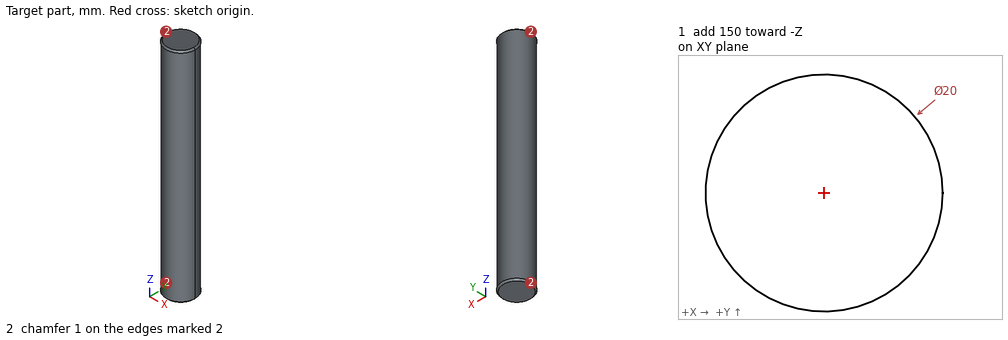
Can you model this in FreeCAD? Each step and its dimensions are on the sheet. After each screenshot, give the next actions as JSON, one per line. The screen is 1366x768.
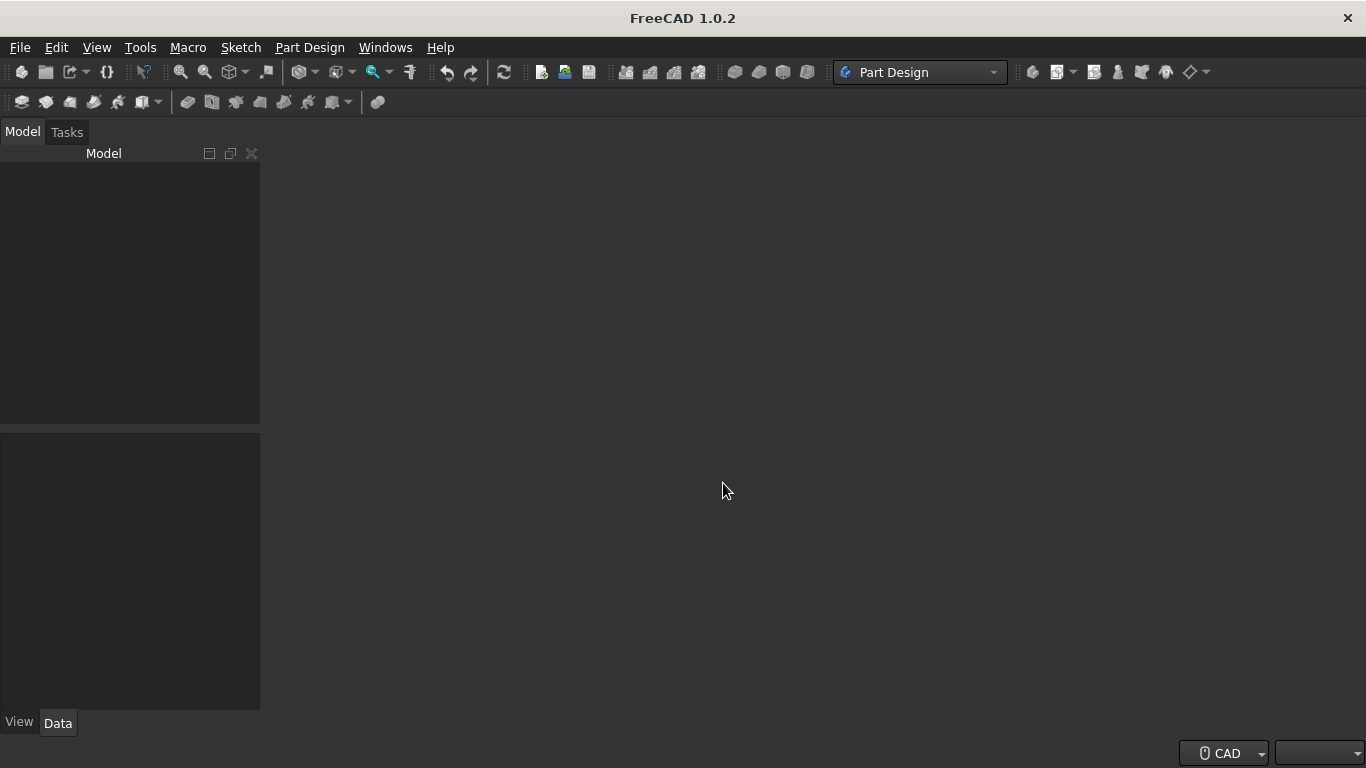
{"action": "key", "text": "ctrl+n"}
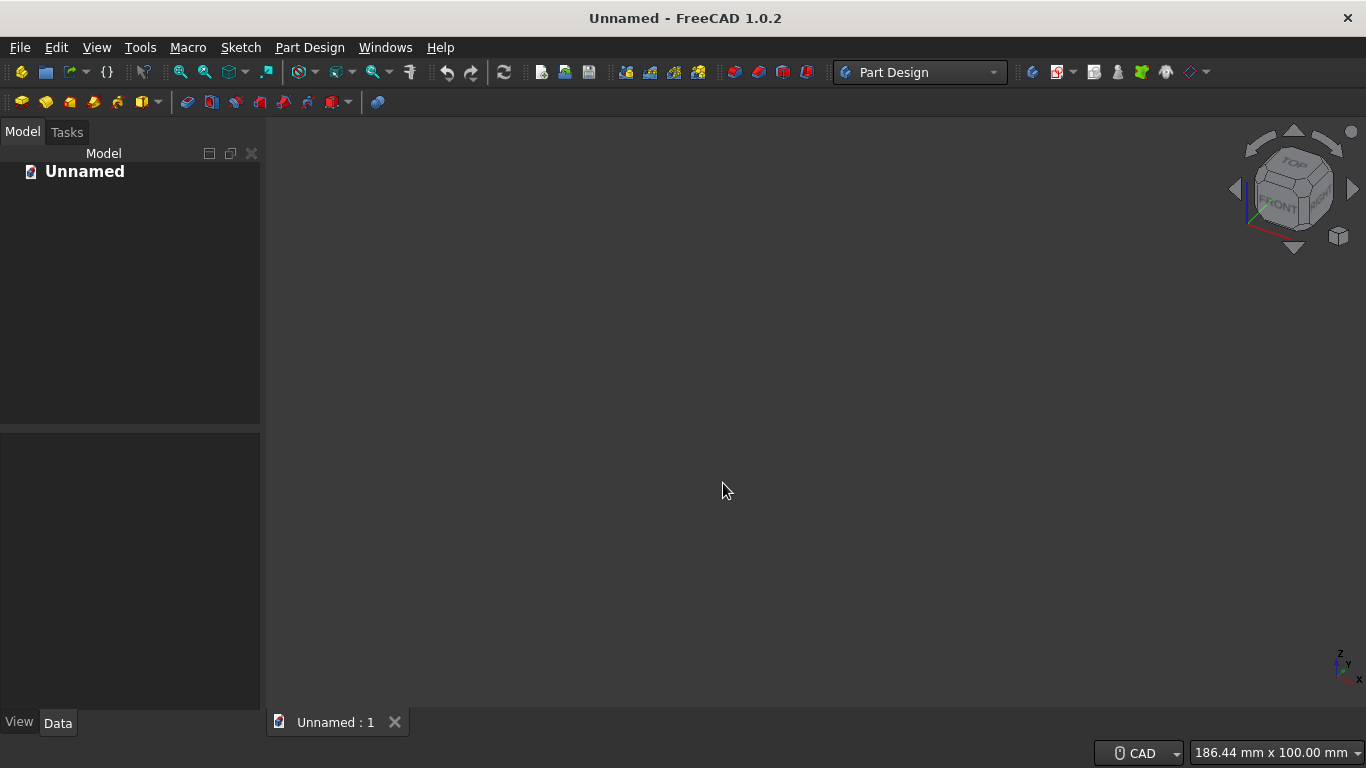
{"action": "left_click", "coordinate": [1058, 72]}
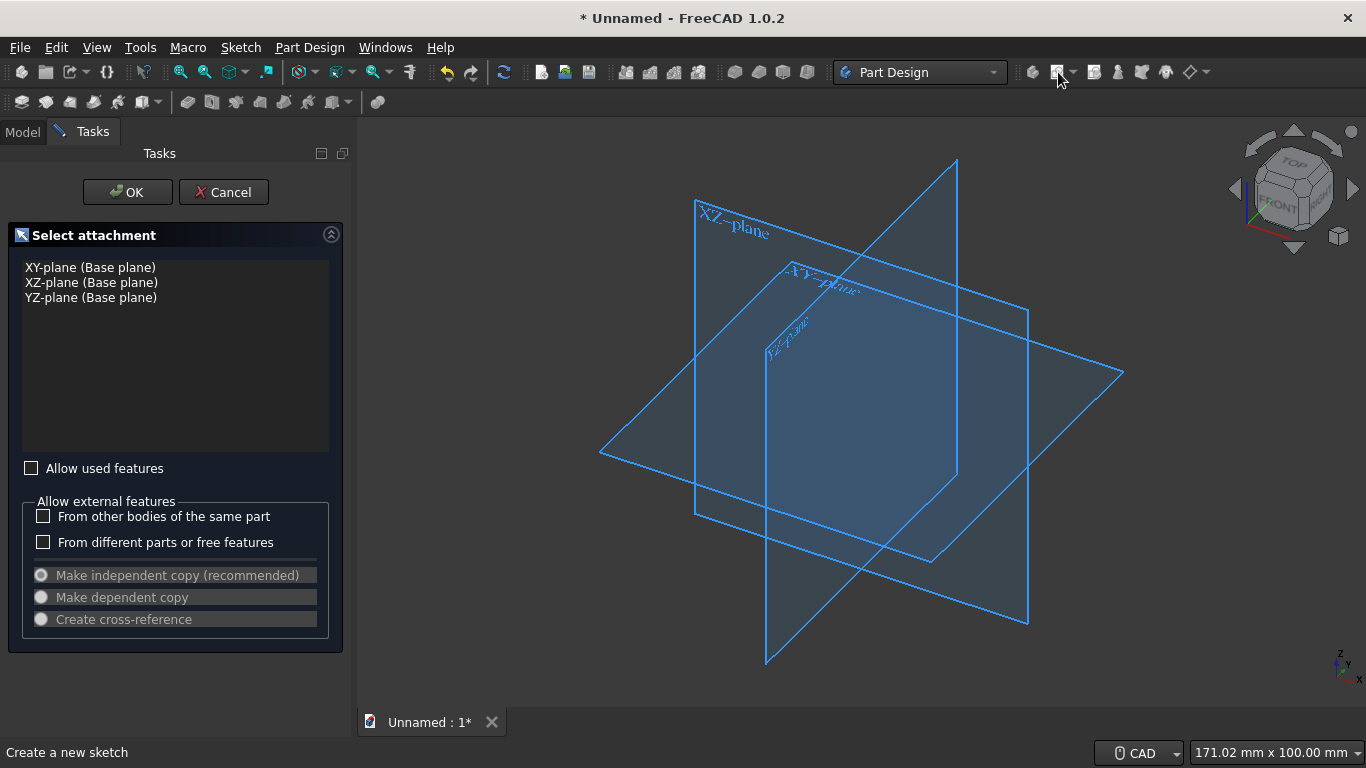
{"action": "left_click", "coordinate": [82, 268]}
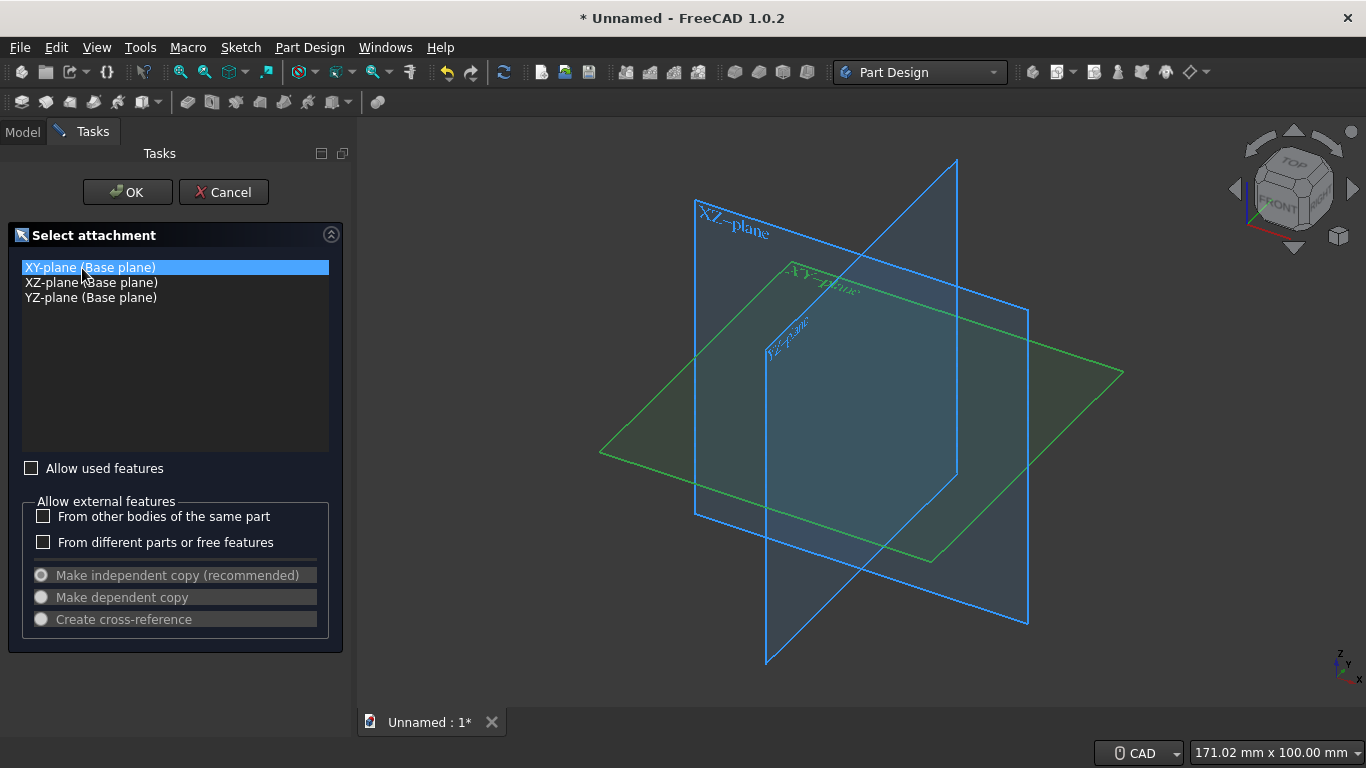
{"action": "left_click", "coordinate": [128, 192]}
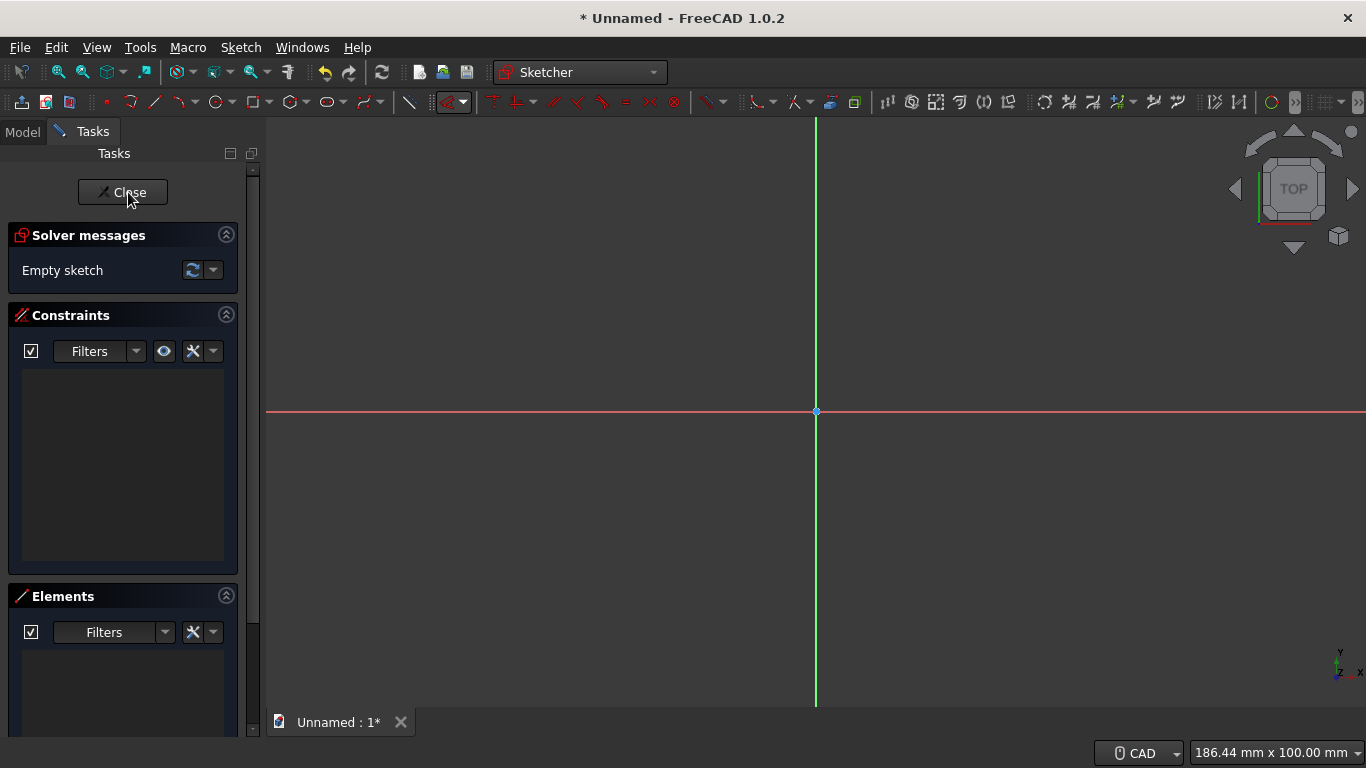
{"action": "scroll", "coordinate": [846, 412], "scroll_direction": "up", "scroll_amount": 6}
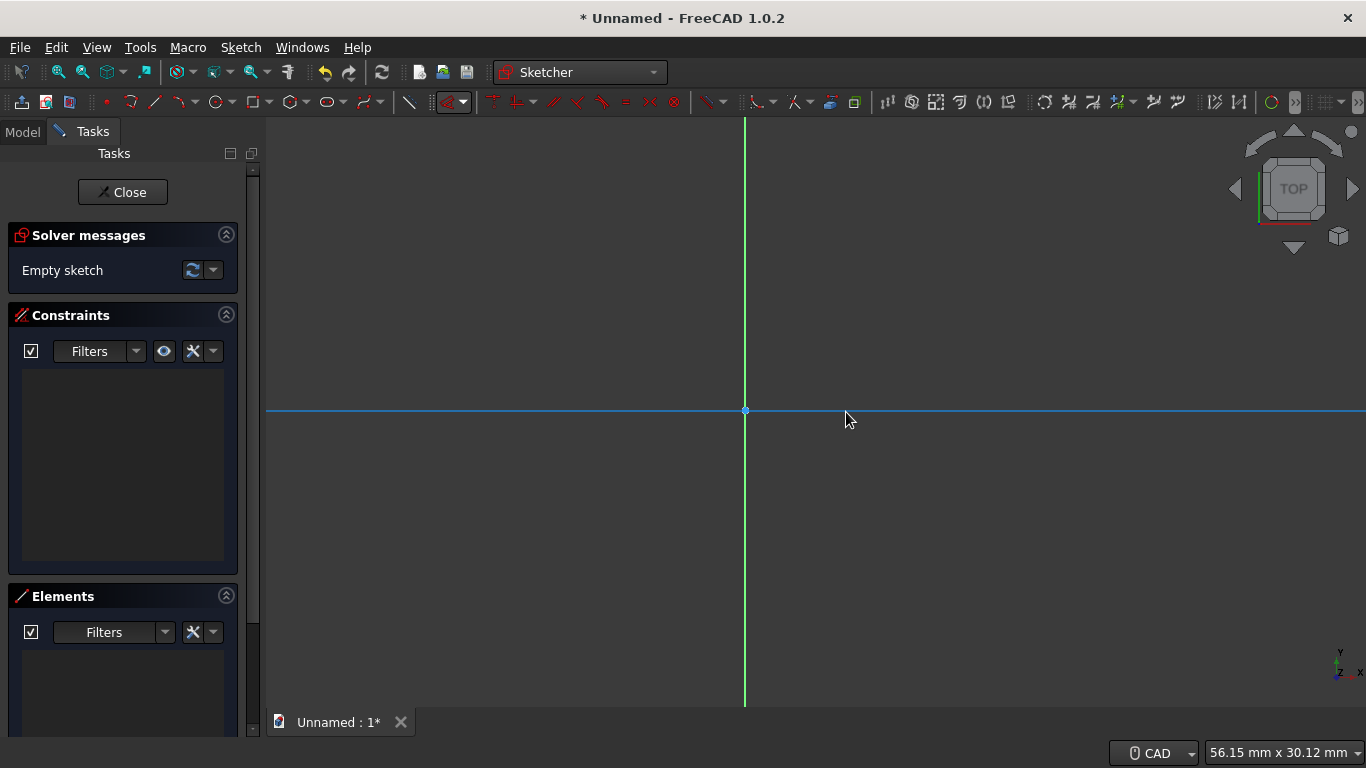
{"action": "key", "text": "g c"}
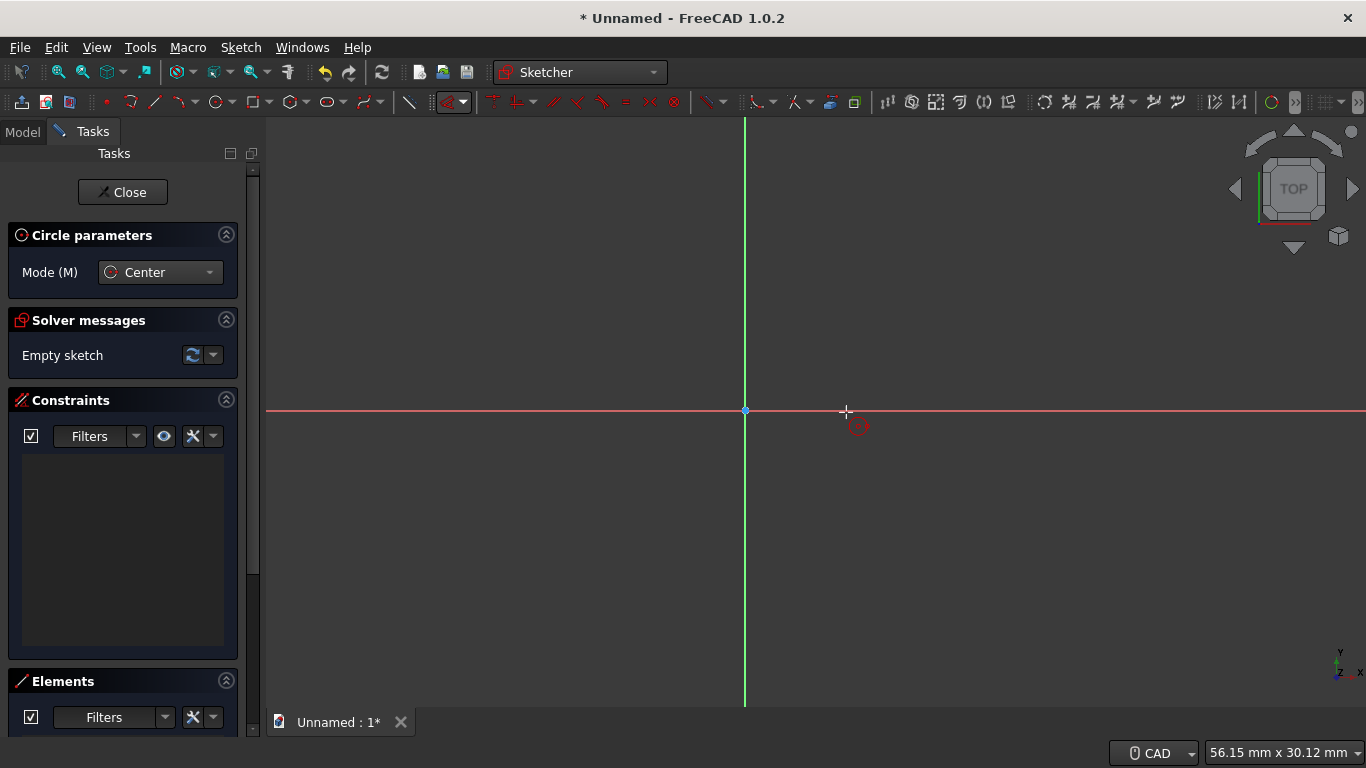
{"action": "left_click", "coordinate": [745, 411]}
{"action": "left_click", "coordinate": [884, 272]}
{"action": "key", "text": "Escape"}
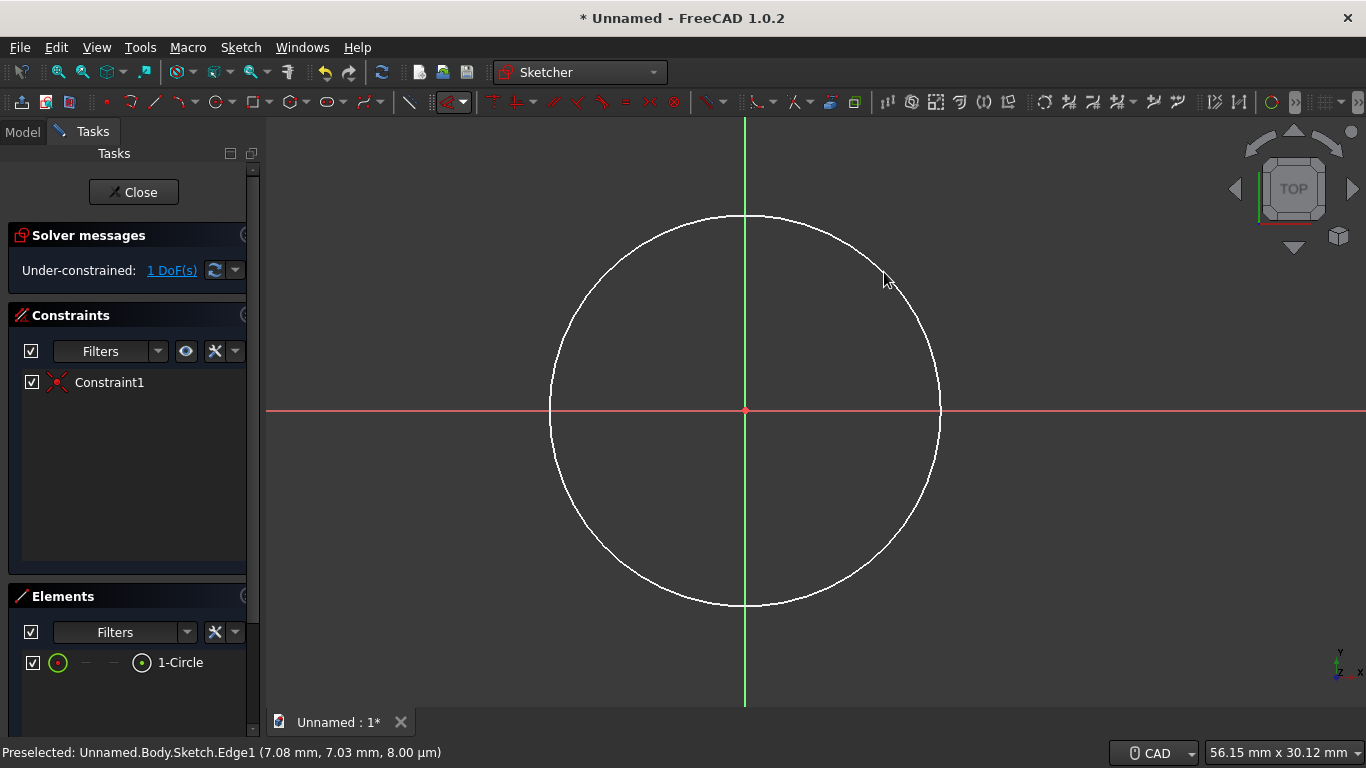
{"action": "left_click", "coordinate": [448, 102]}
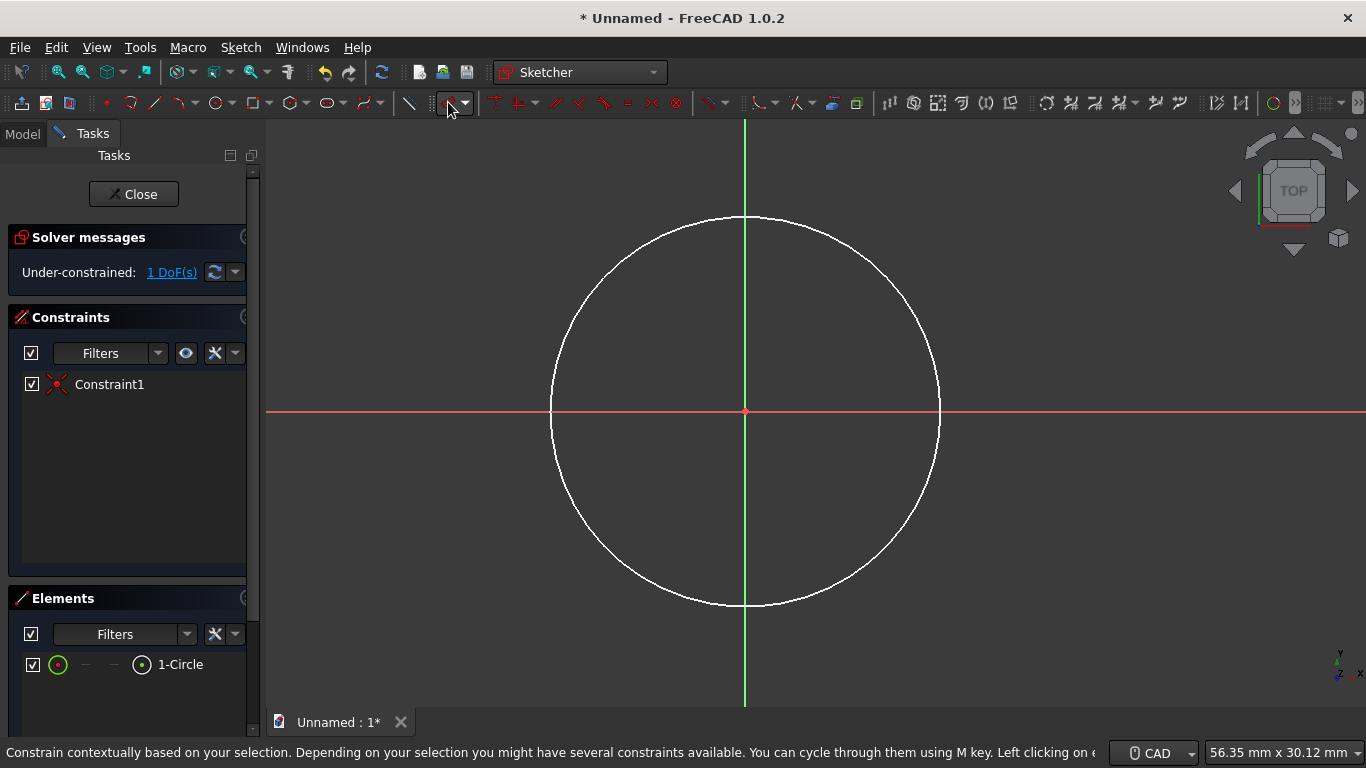
{"action": "left_click", "coordinate": [883, 274]}
{"action": "left_click", "coordinate": [906, 251]}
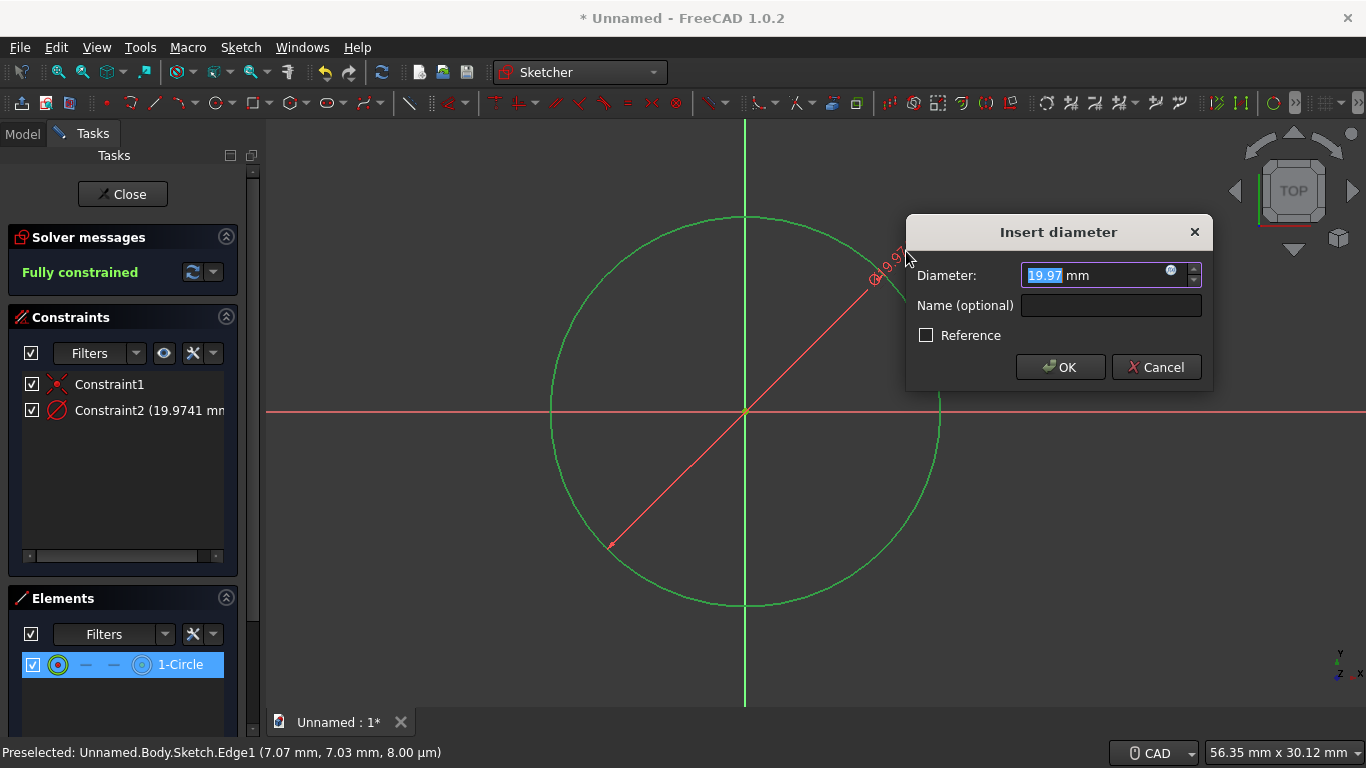
{"action": "type", "text": "20"}
{"action": "key", "text": "Return"}
{"action": "key", "text": "Escape"}